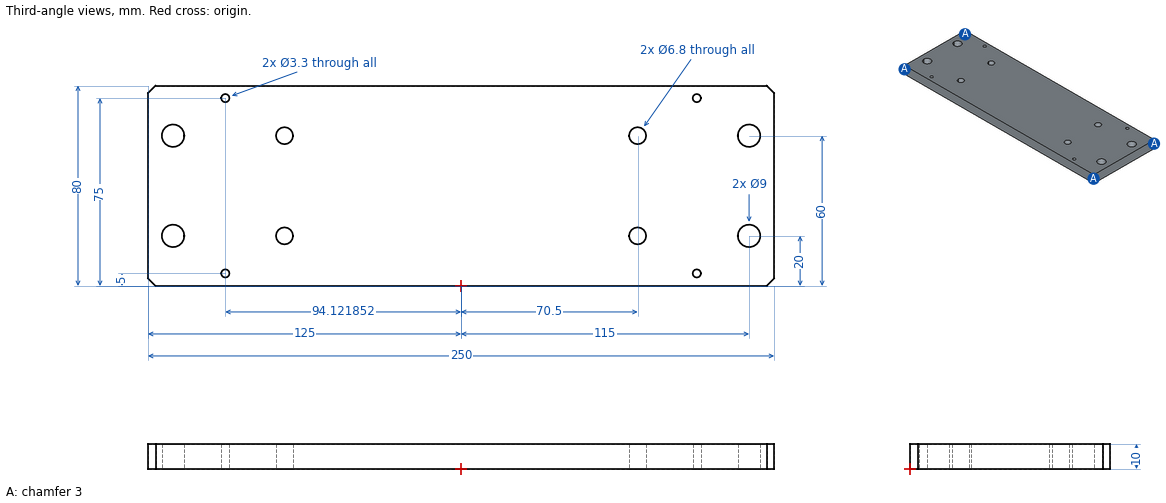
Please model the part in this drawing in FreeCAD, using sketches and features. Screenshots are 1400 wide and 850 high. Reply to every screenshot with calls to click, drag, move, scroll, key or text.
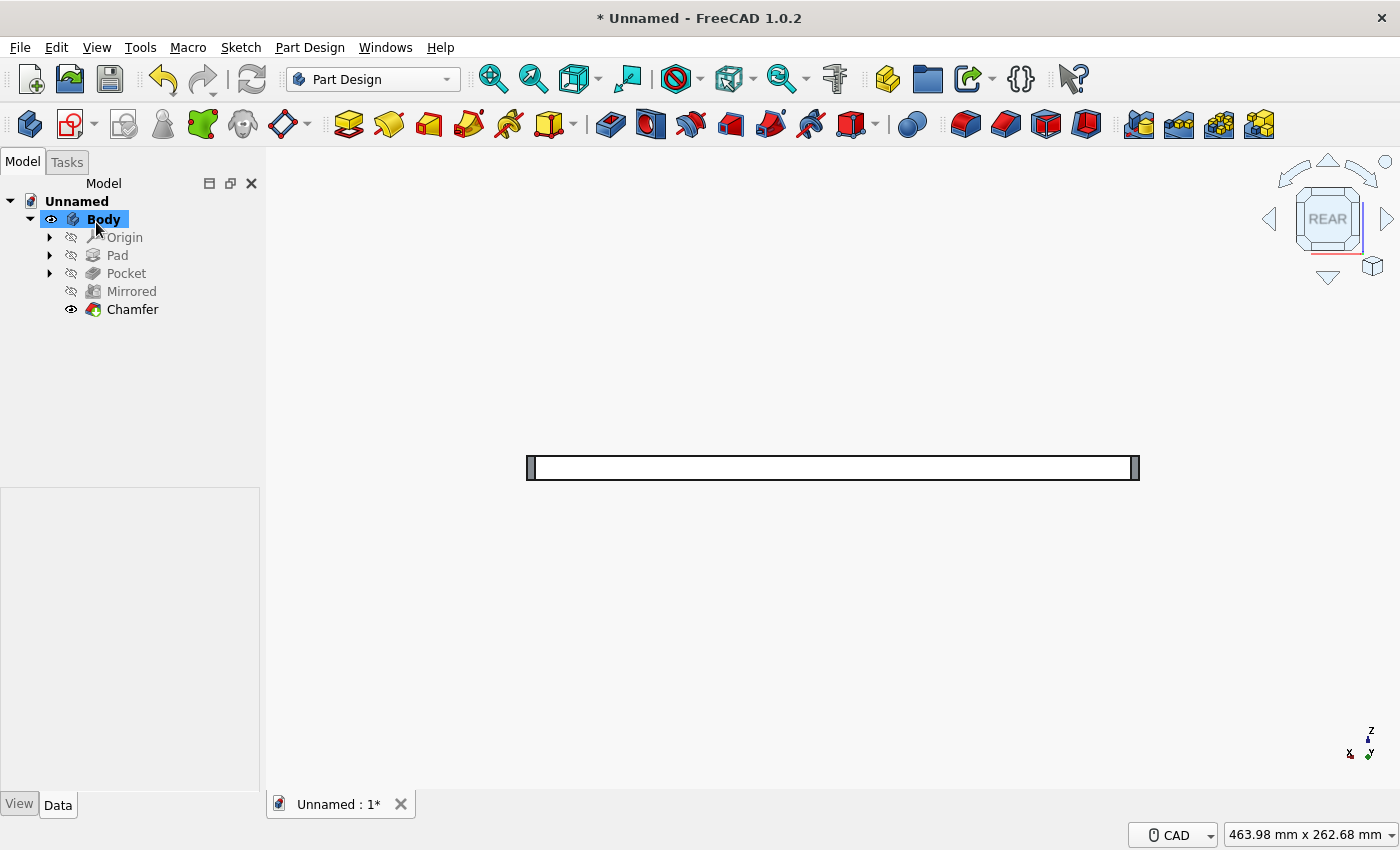
key(0)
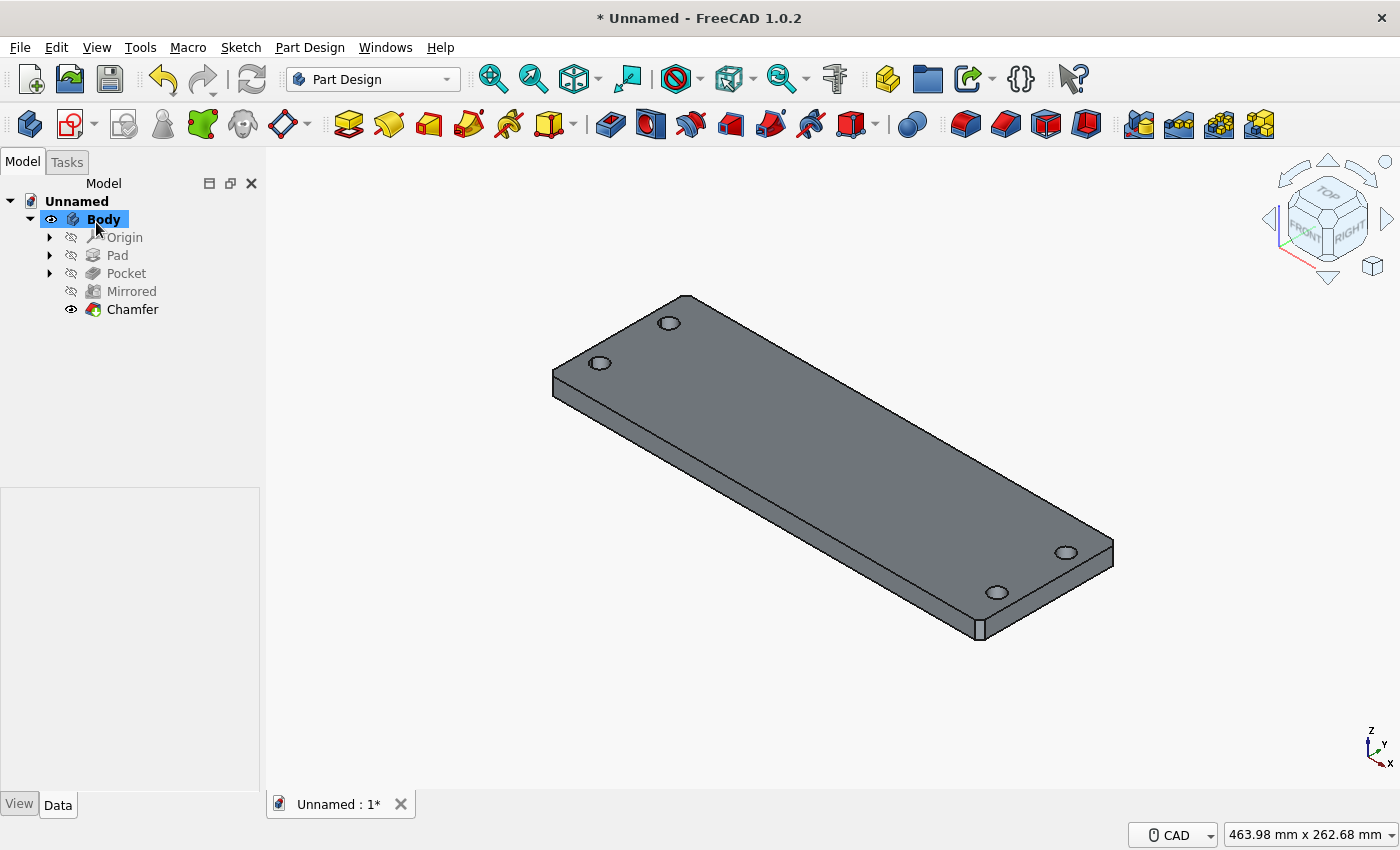
click(956, 528)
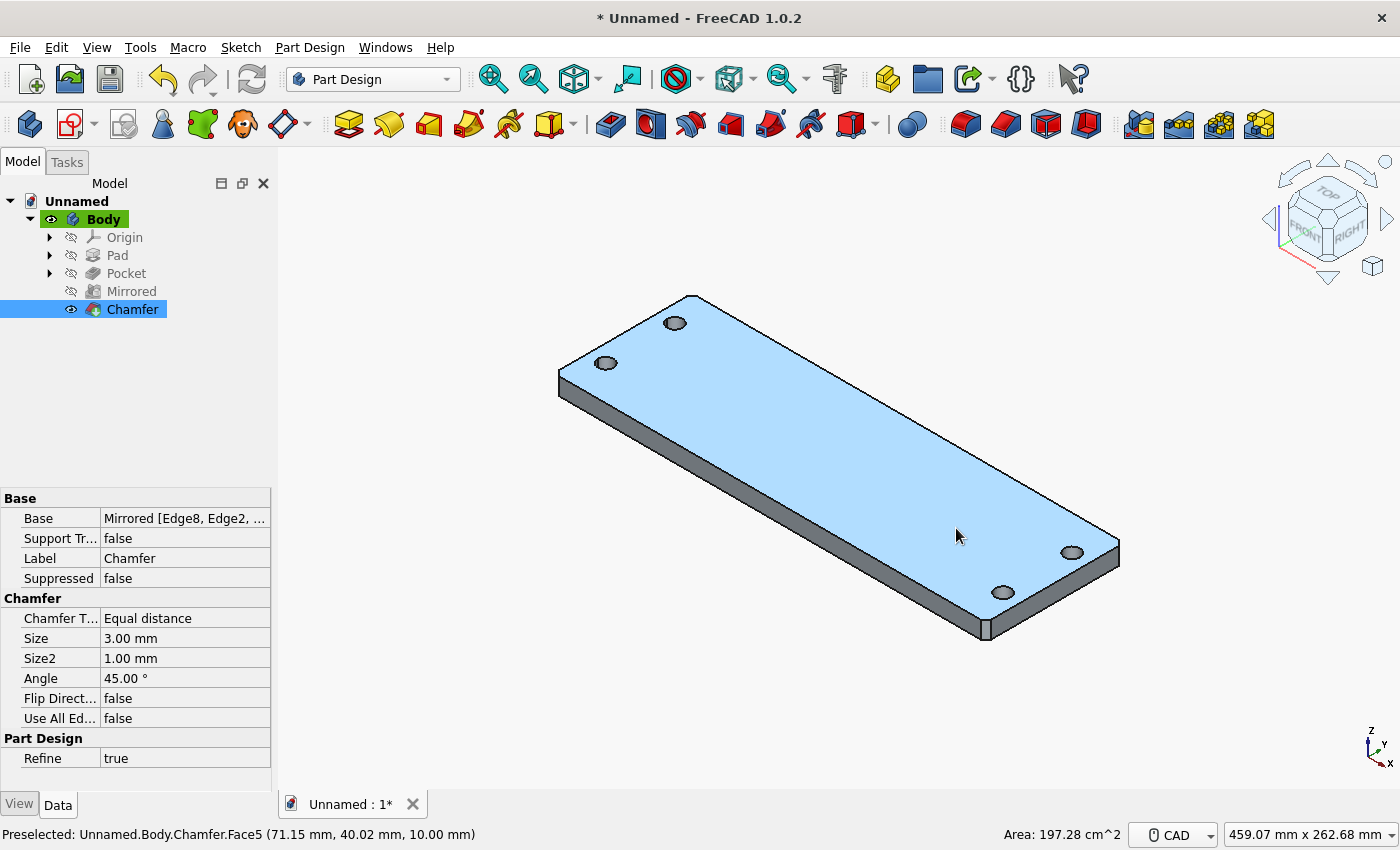
click(70, 124)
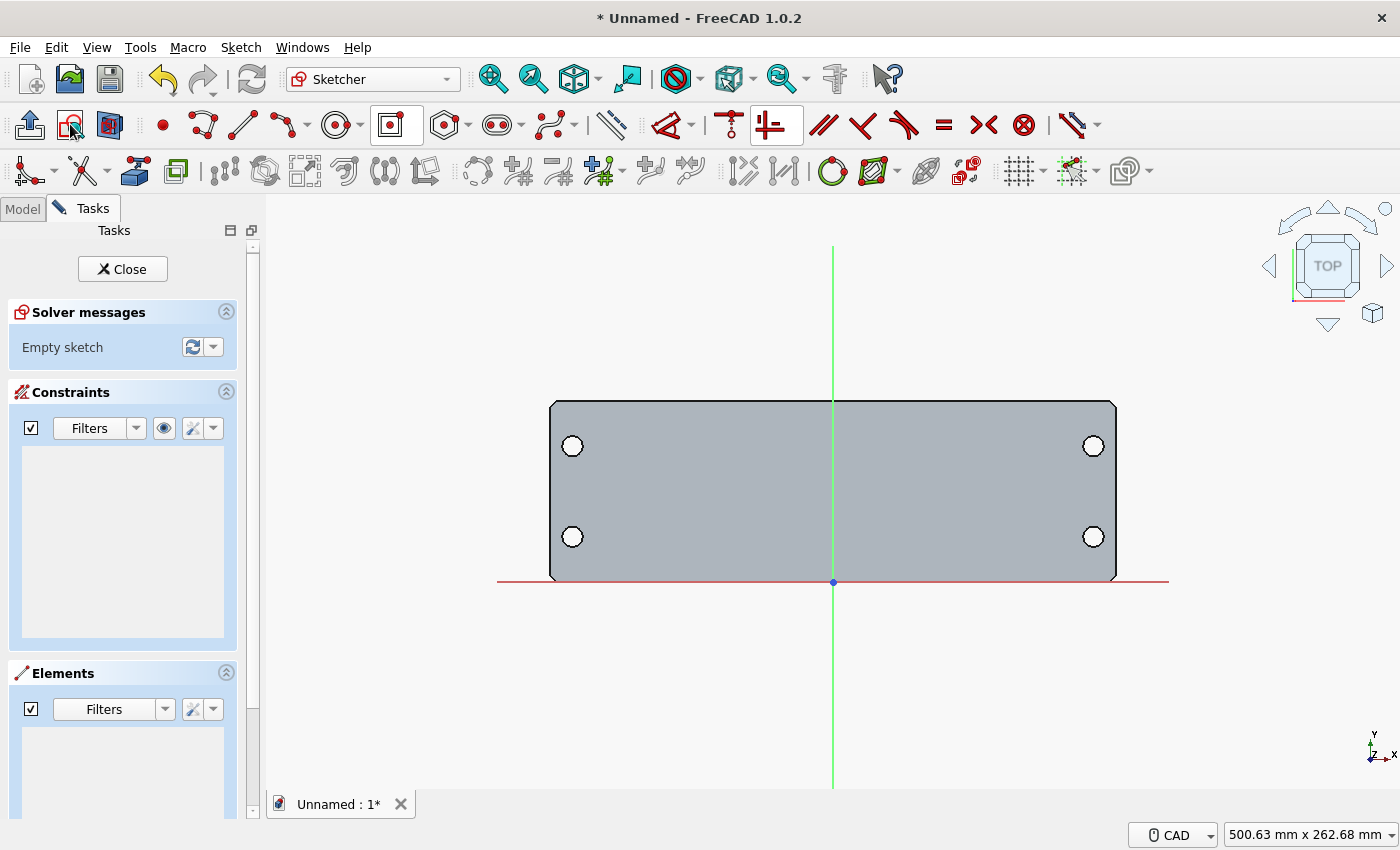
scroll(1005, 521, up, 5)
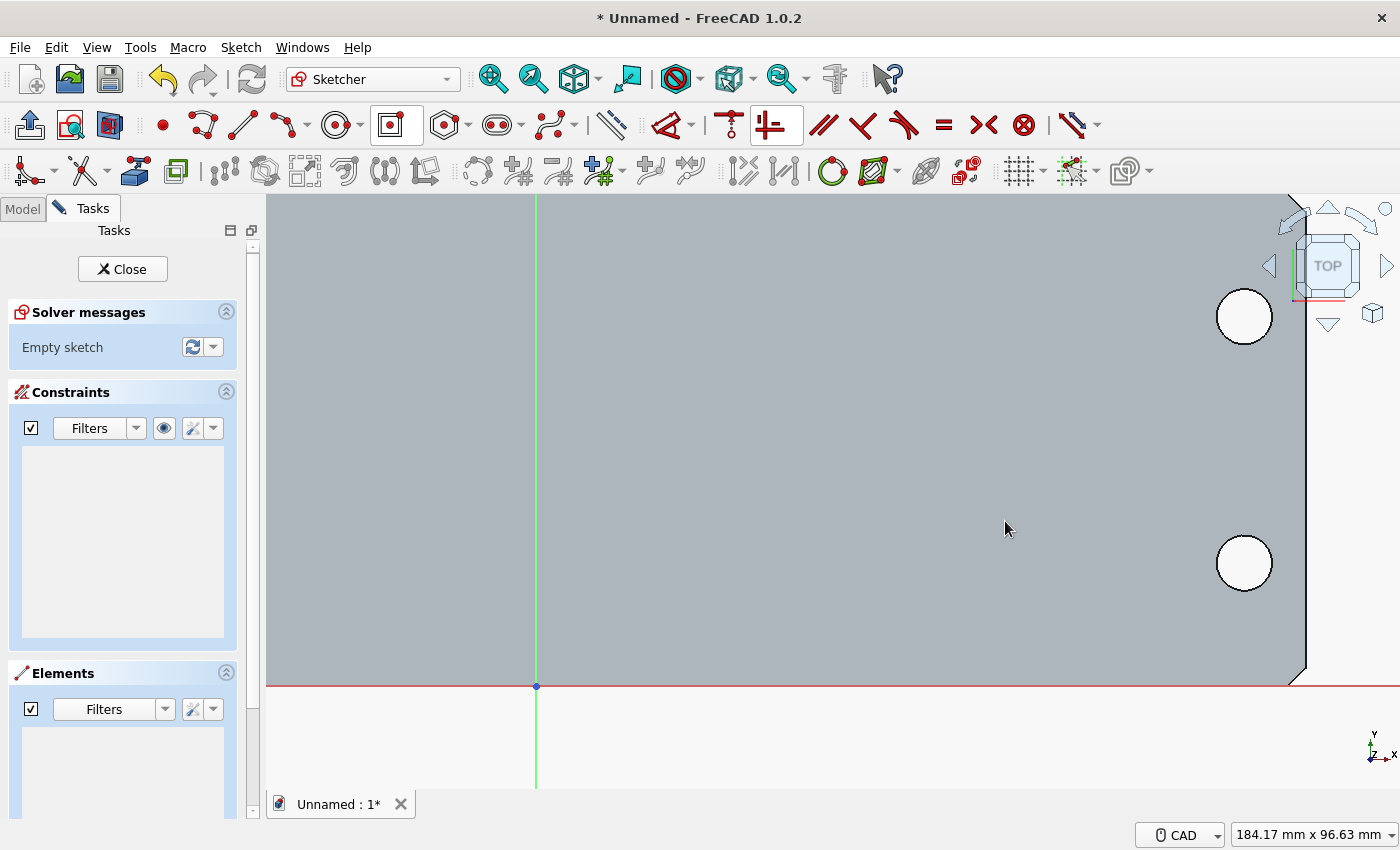
click(336, 126)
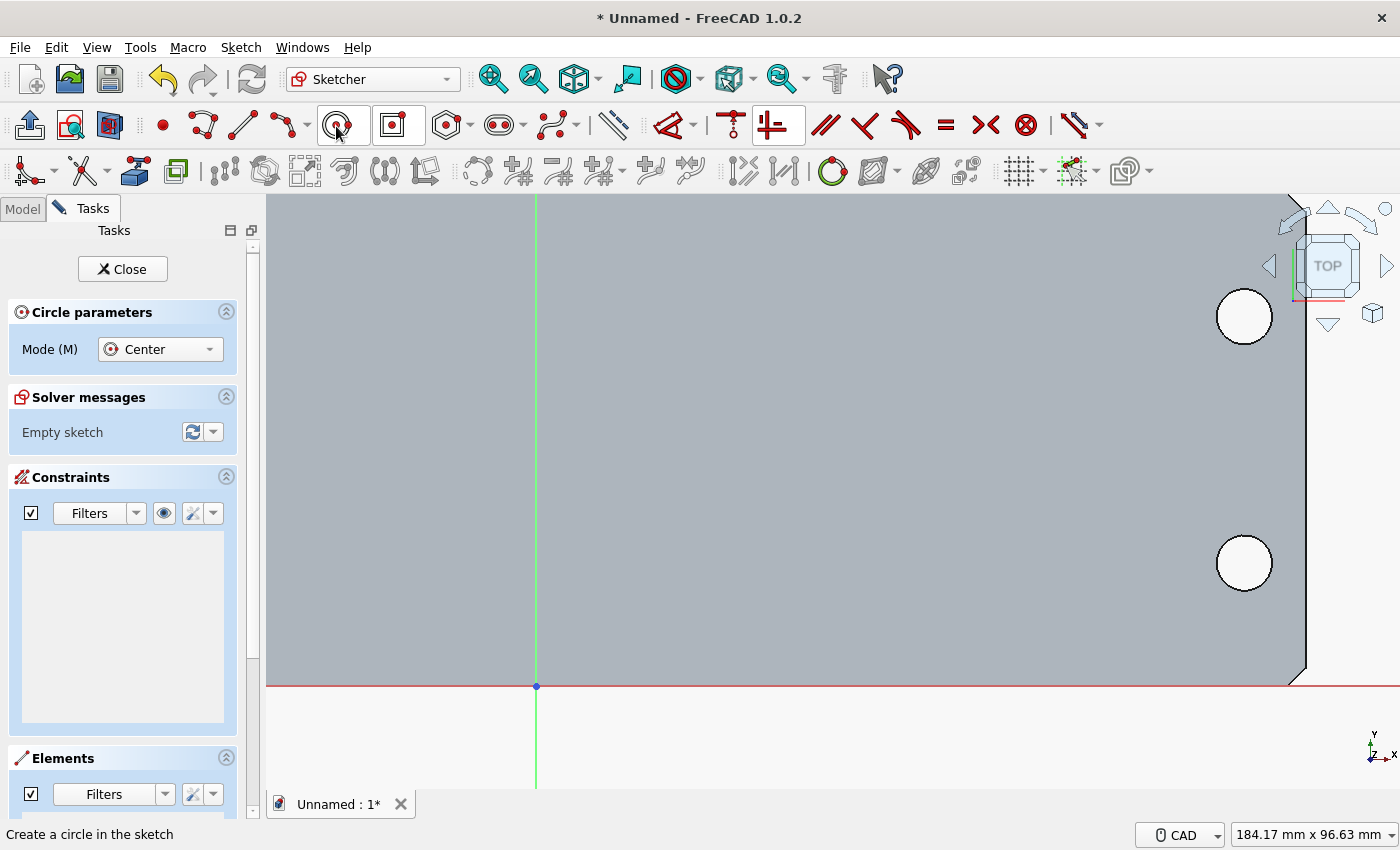
click(970, 317)
move(985, 302)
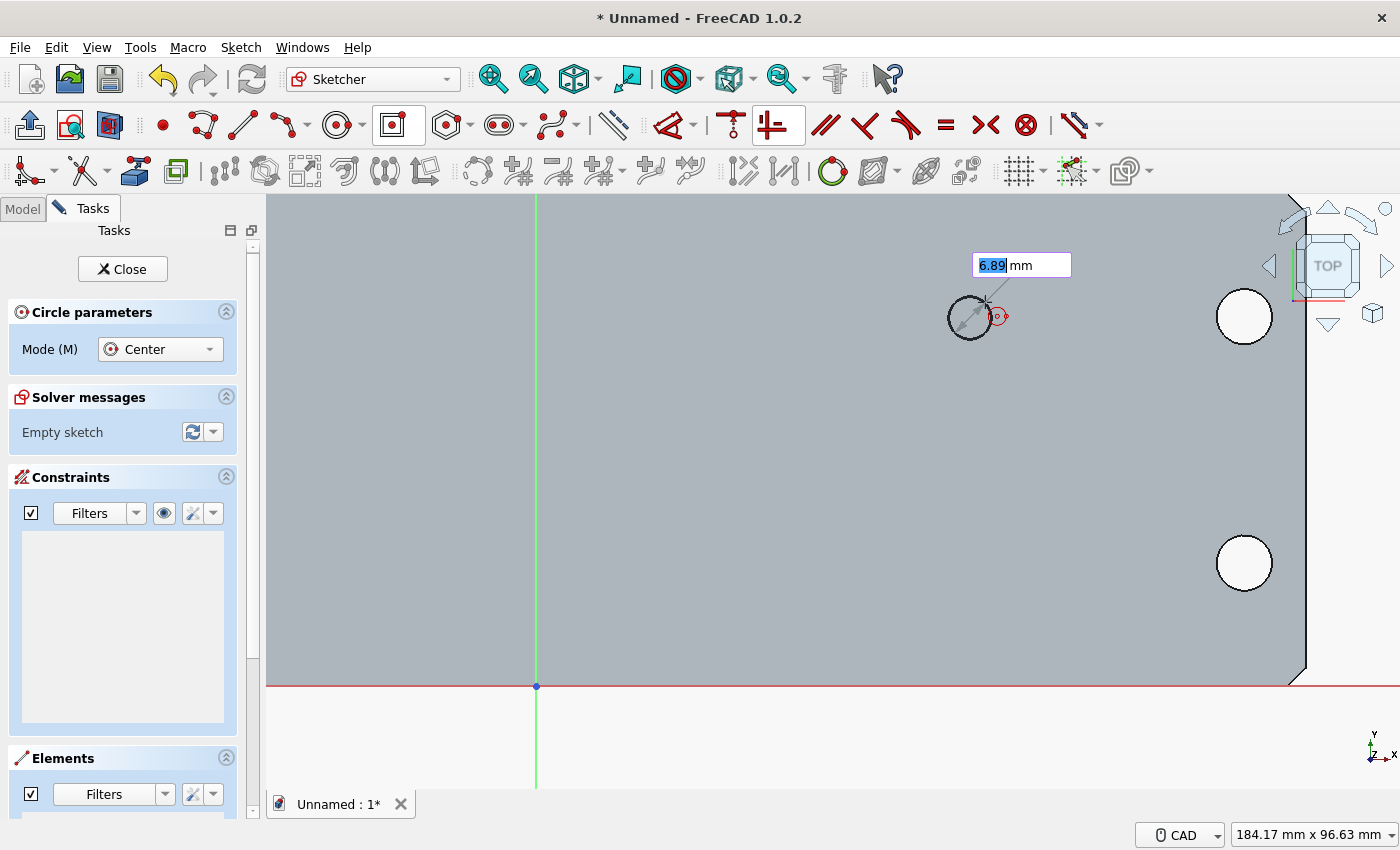
text(6.8)
key(Return)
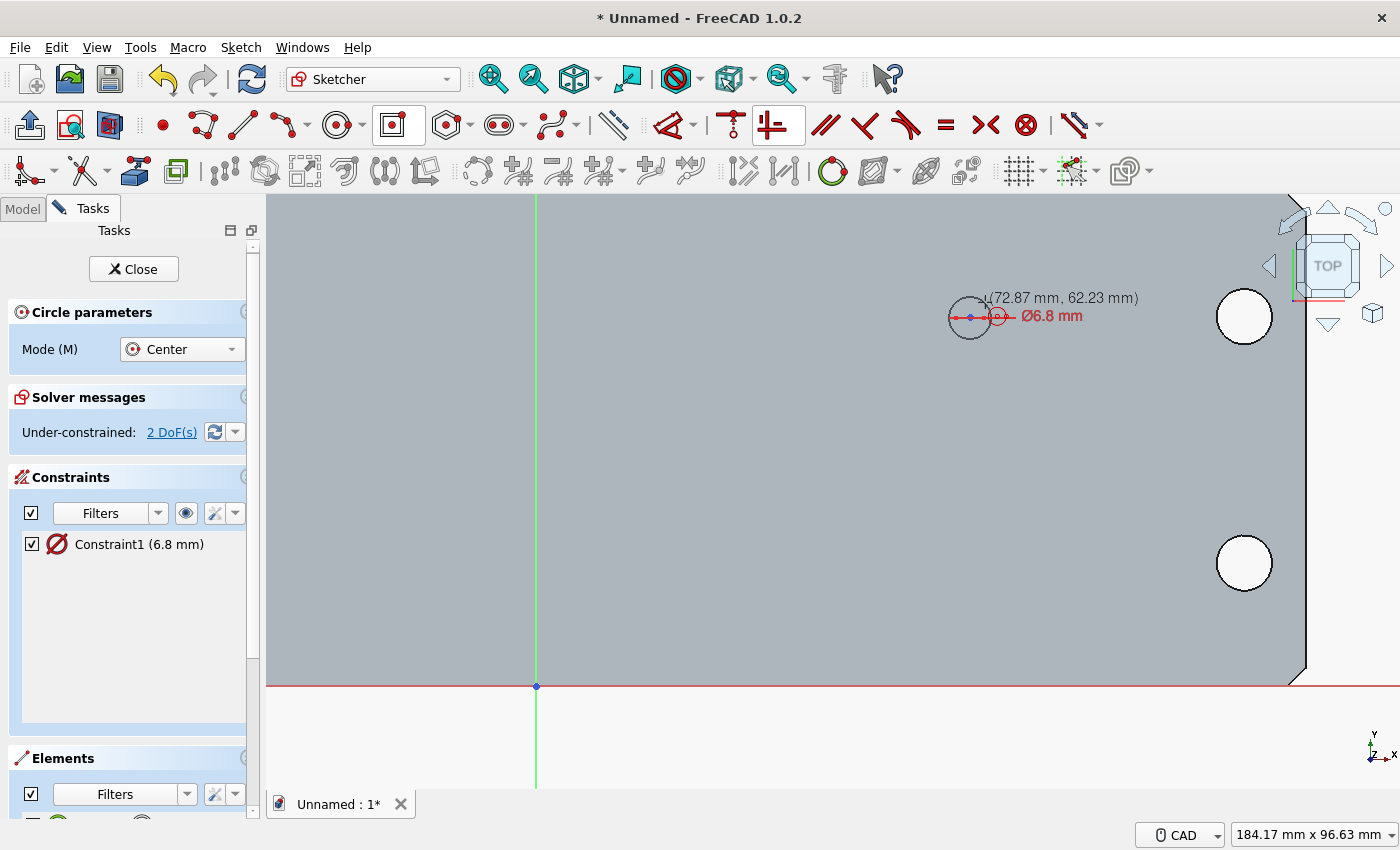
click(970, 563)
move(985, 548)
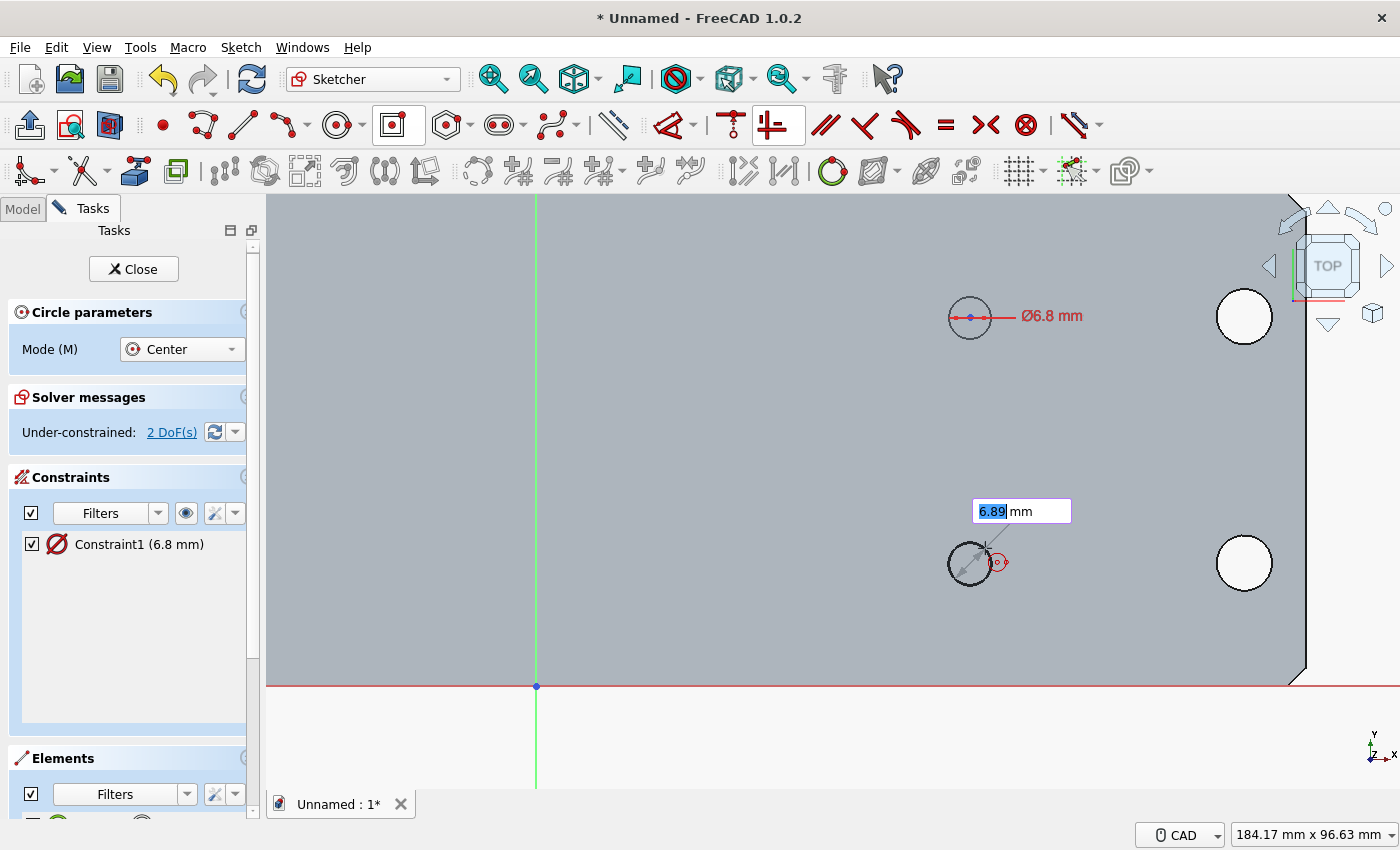
text(6.8)
key(Return)
key(Escape)